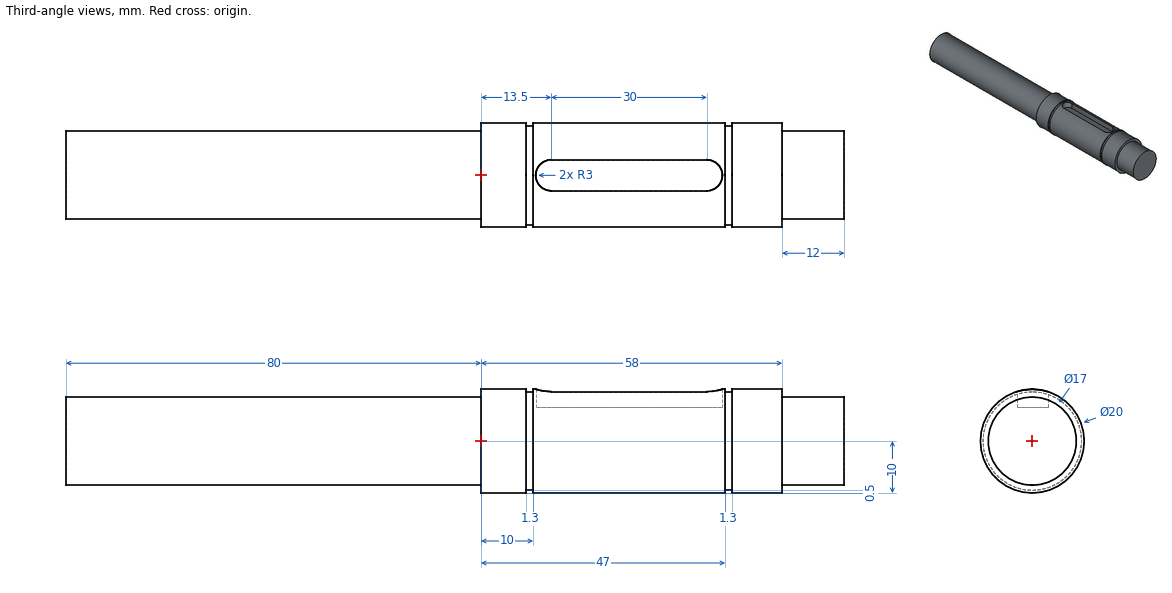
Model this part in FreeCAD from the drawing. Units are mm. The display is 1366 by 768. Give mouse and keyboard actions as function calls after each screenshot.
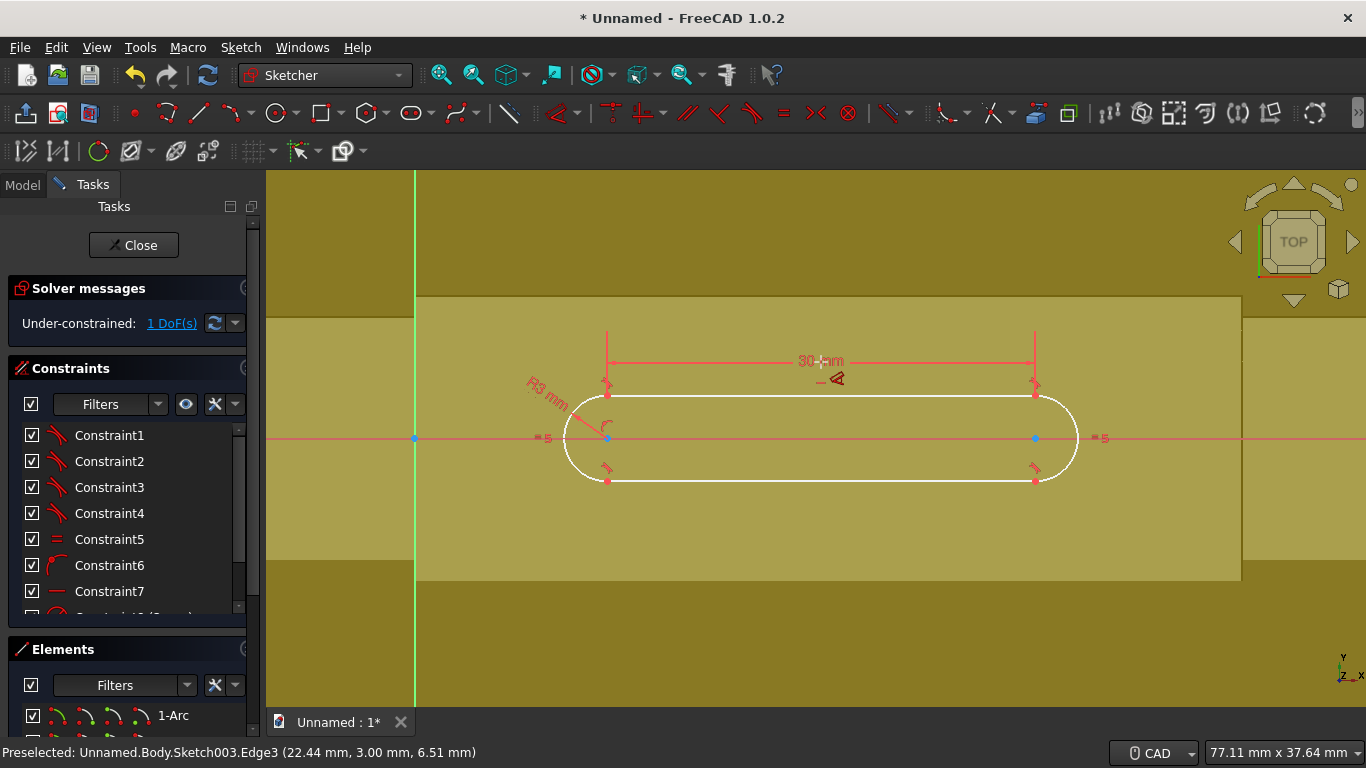
click(607, 396)
click(511, 362)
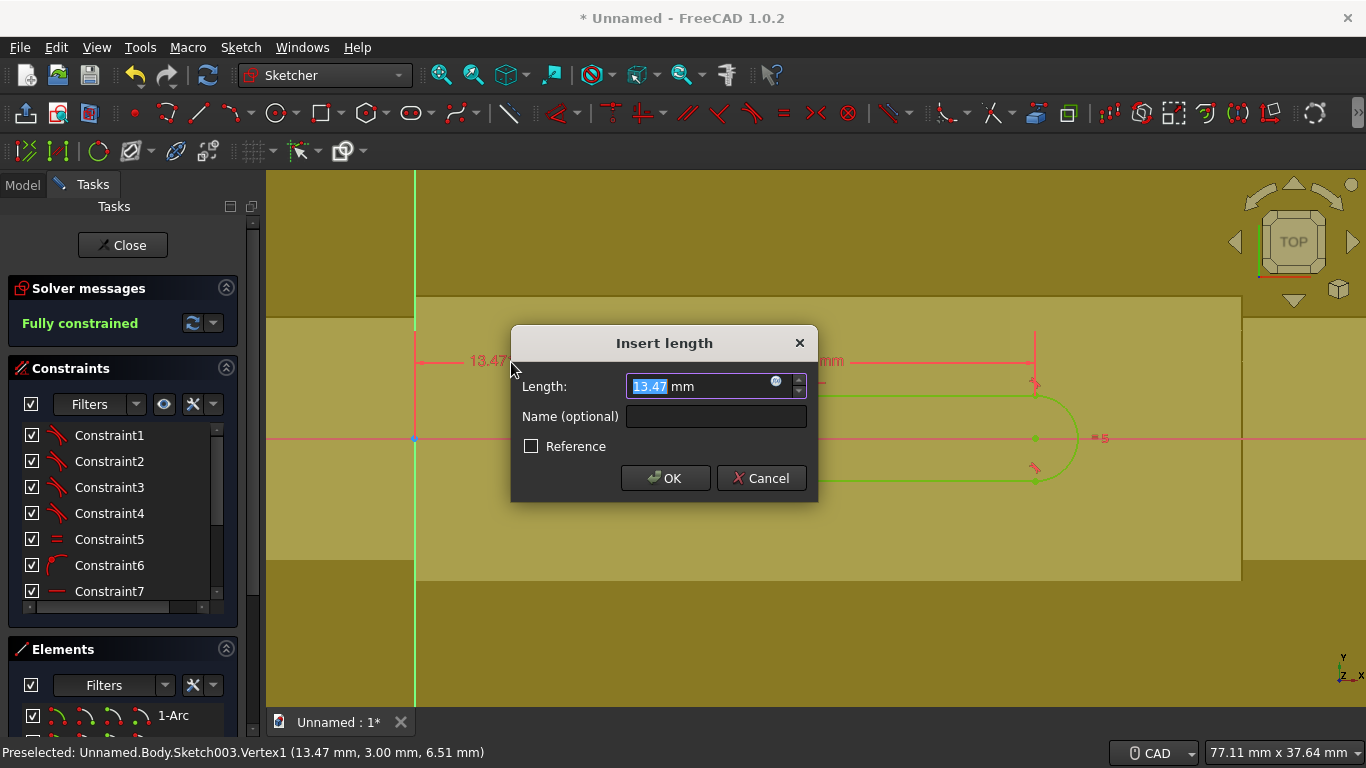
text(13.5)
key(Return)
key(Escape)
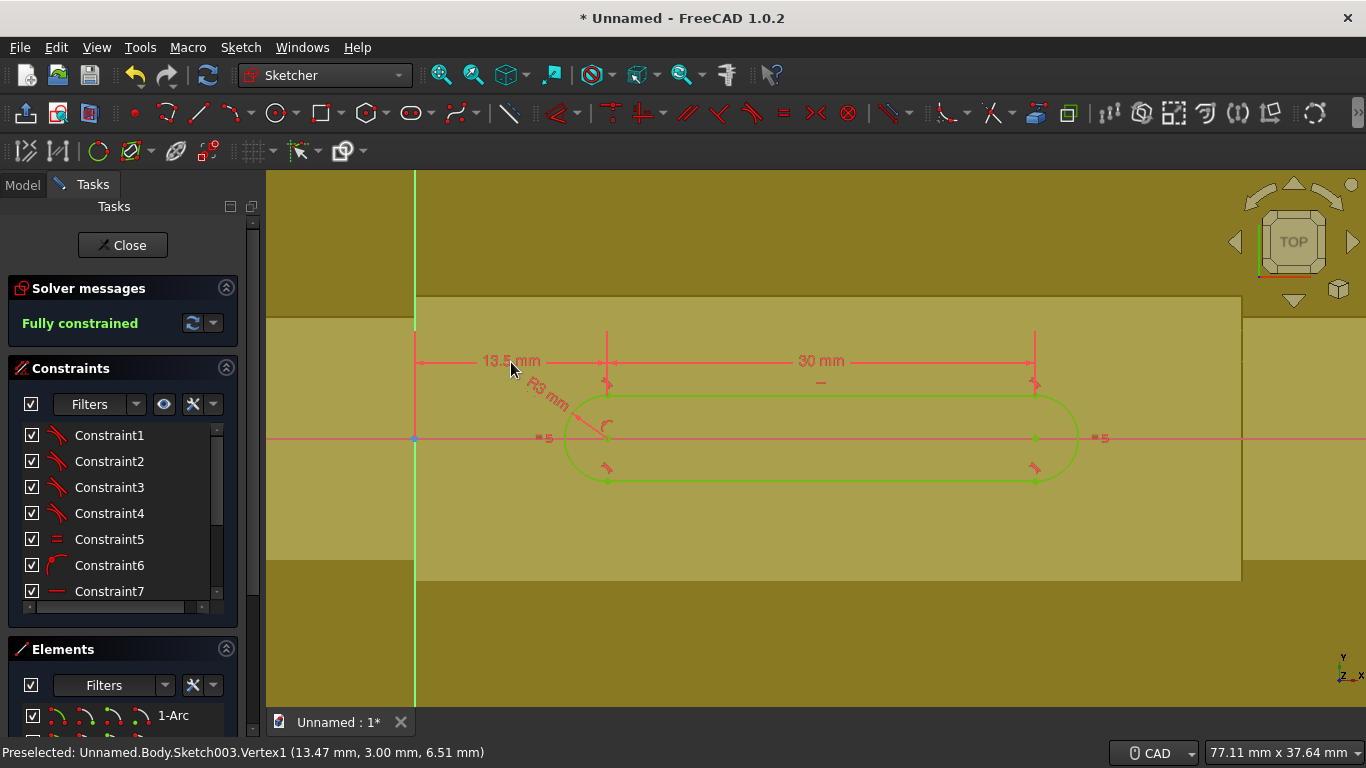
click(123, 245)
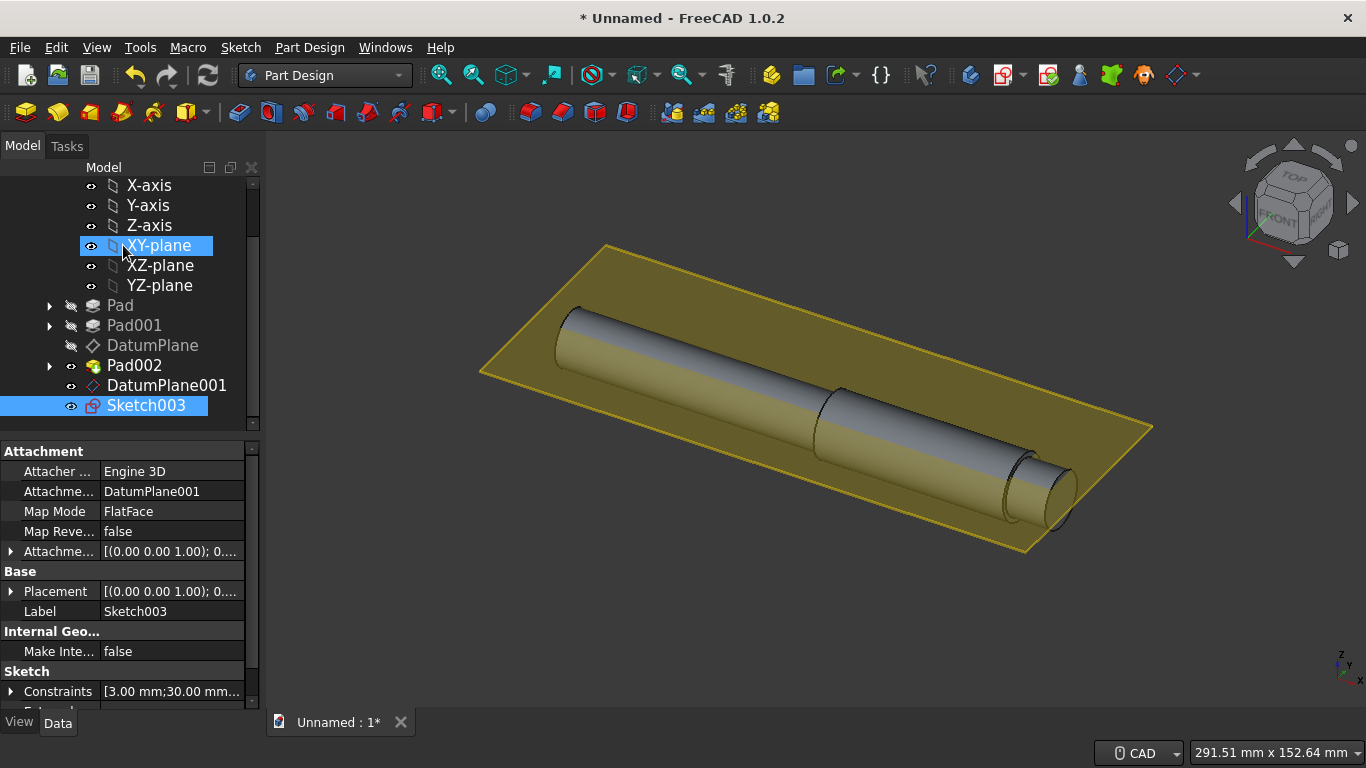
click(240, 112)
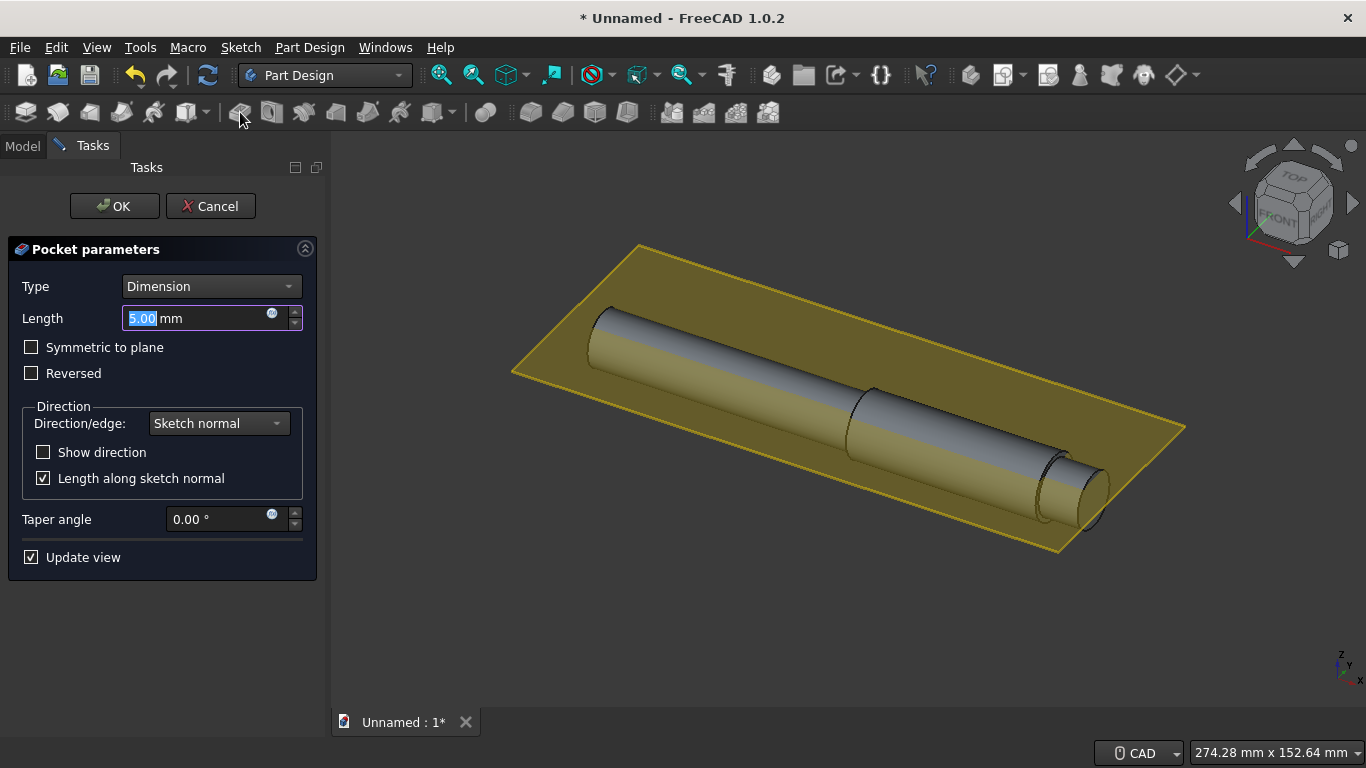
click(212, 286)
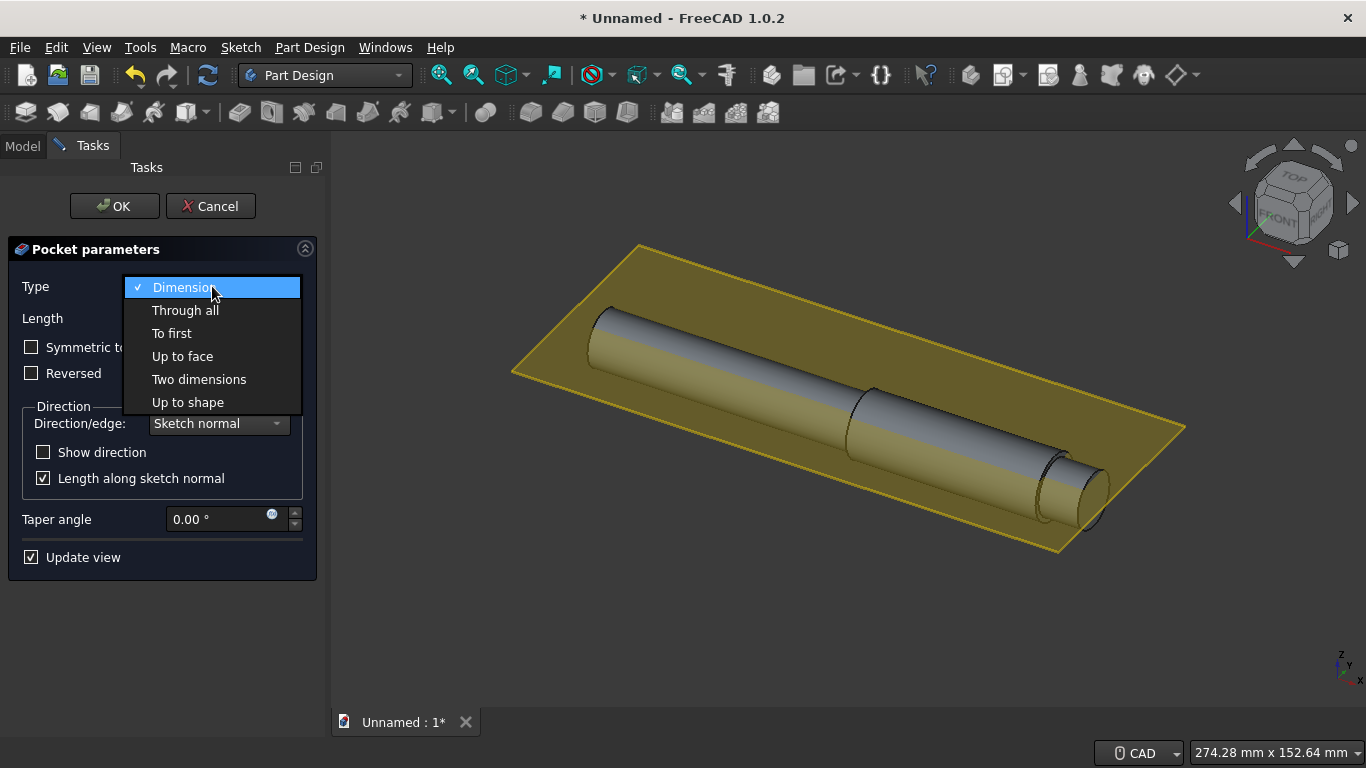
click(212, 310)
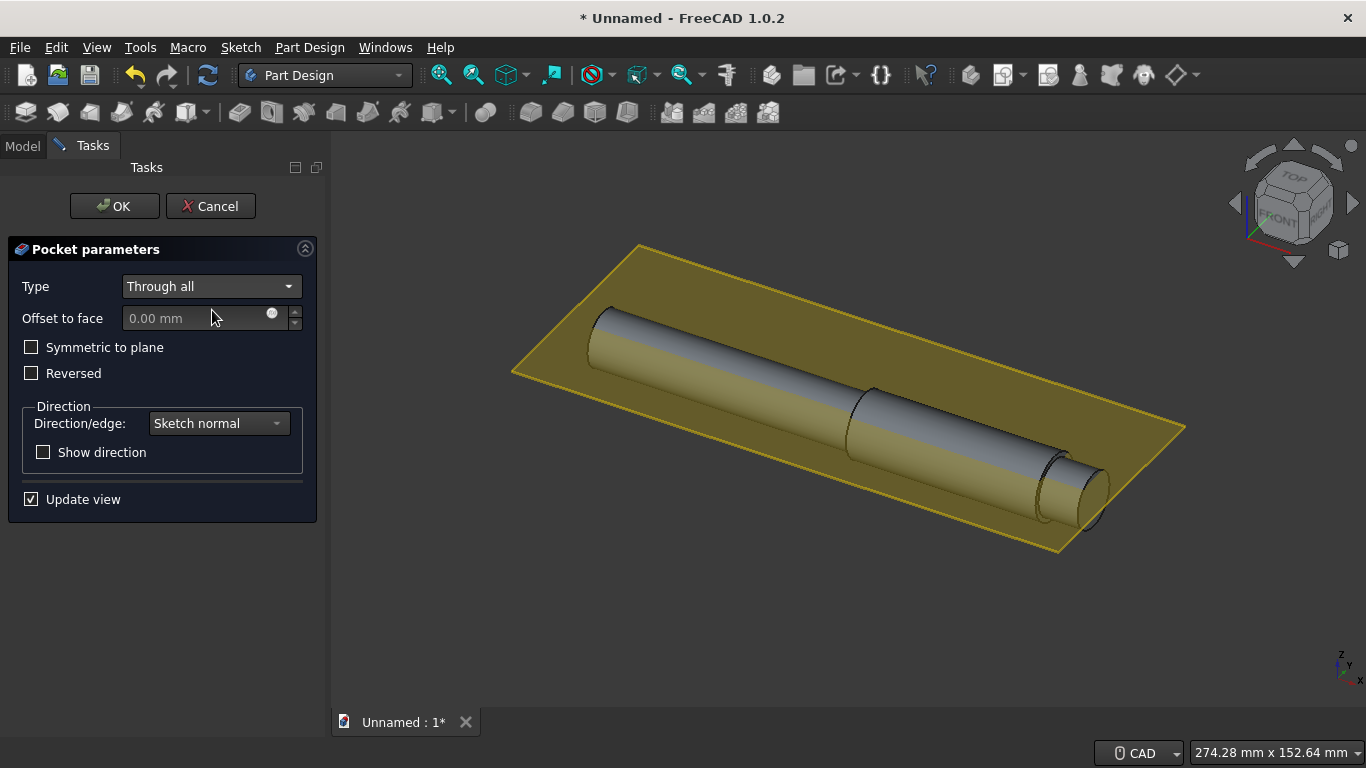
click(30, 373)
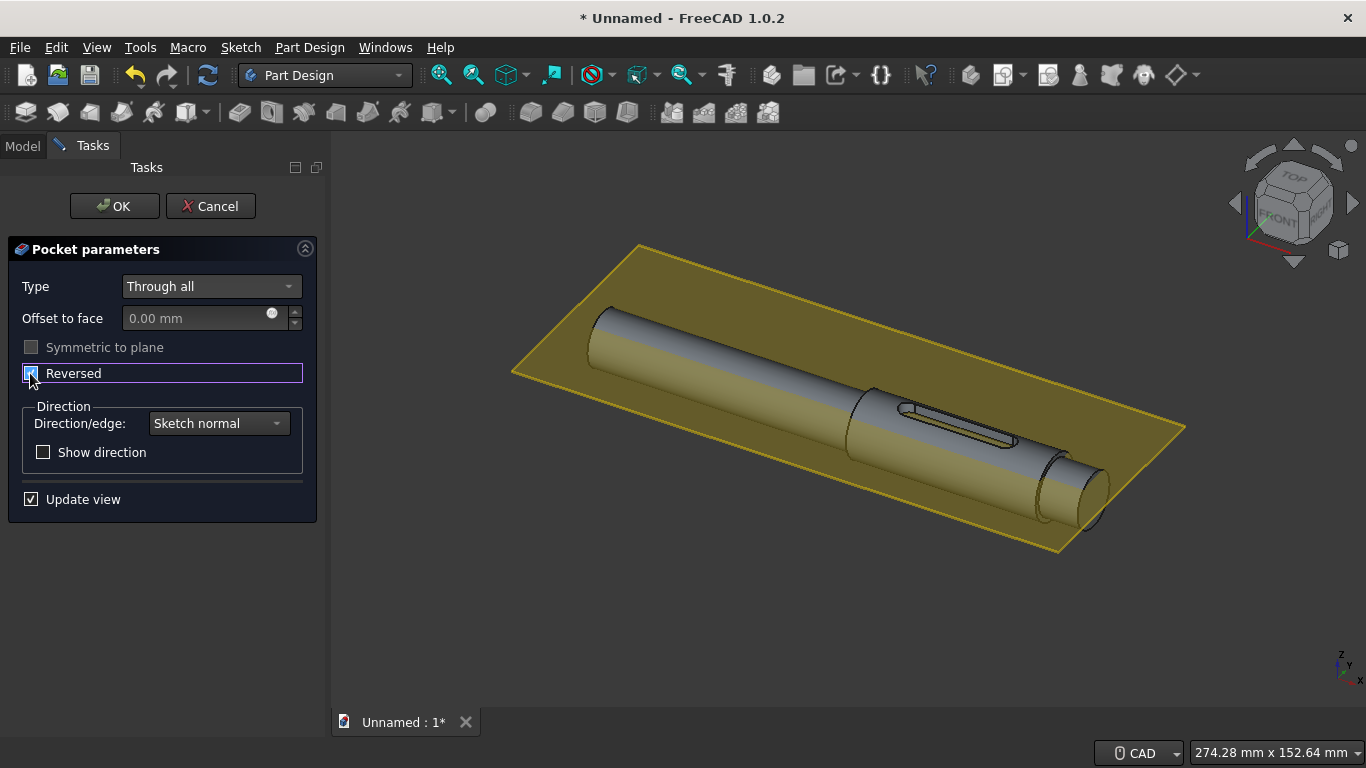
click(115, 206)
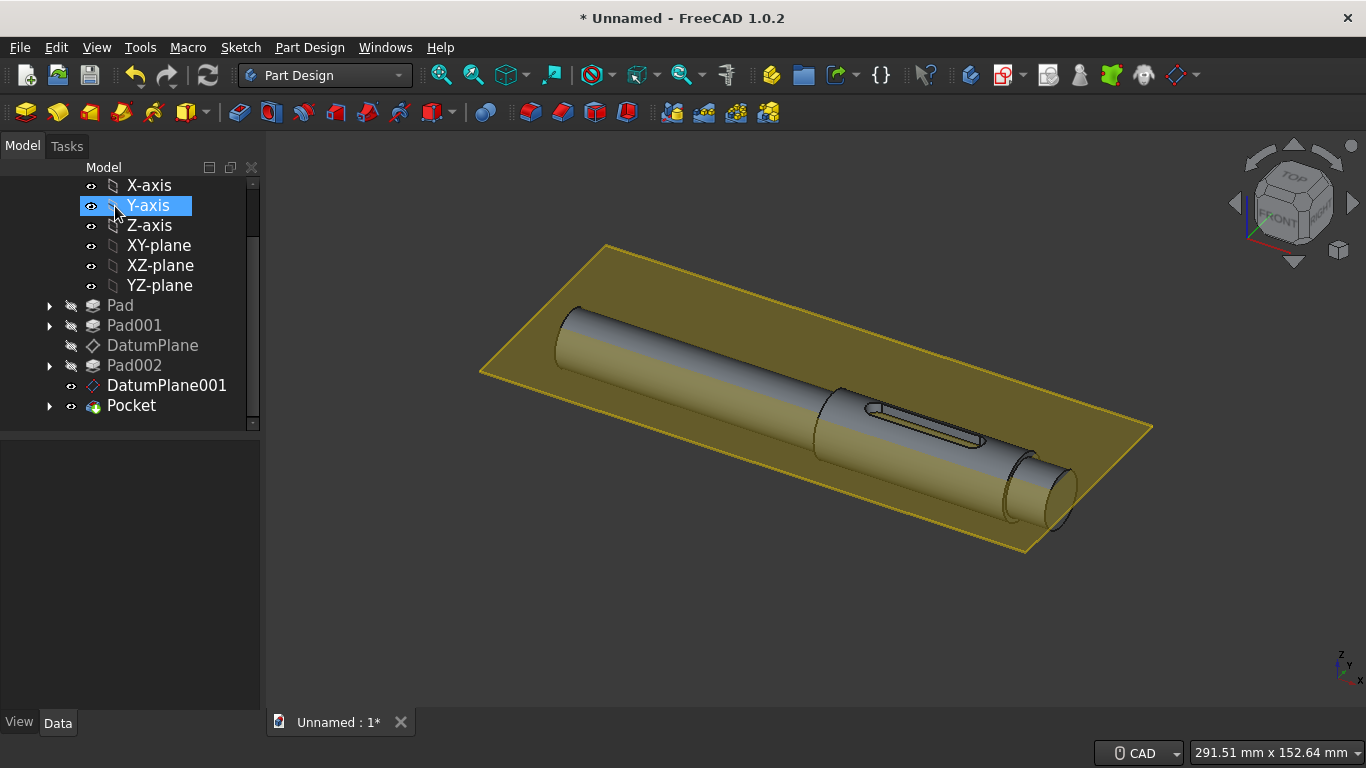
click(116, 386)
key(space)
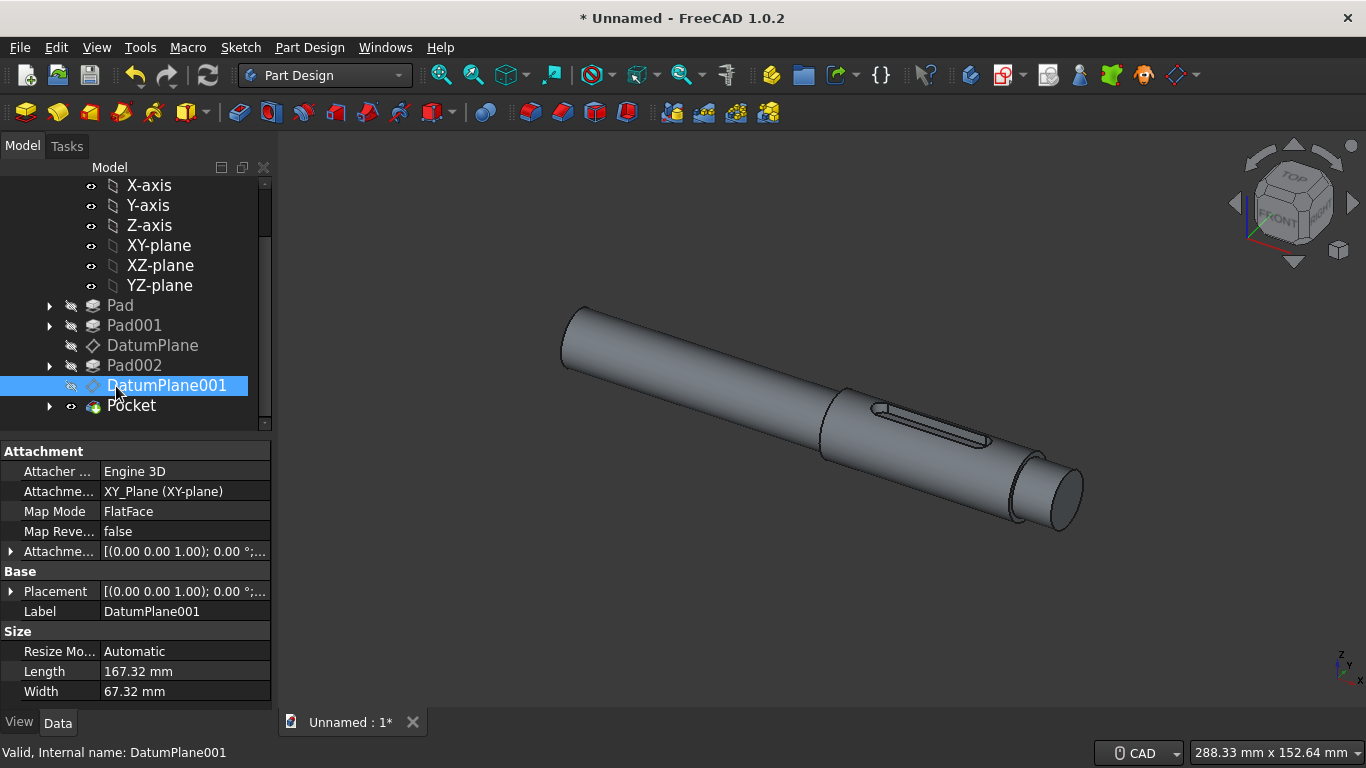
click(318, 667)